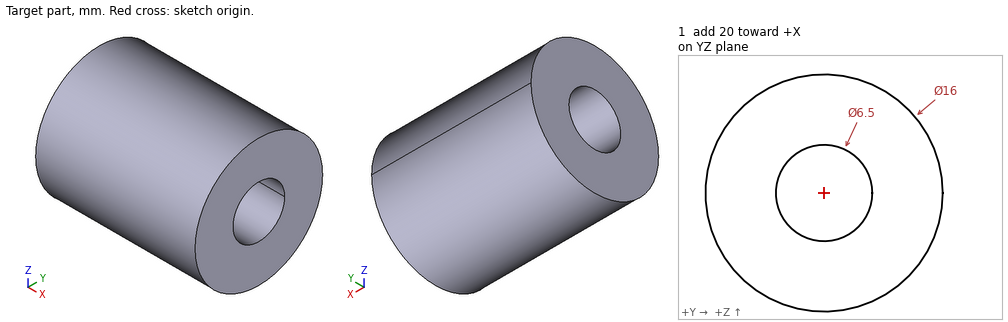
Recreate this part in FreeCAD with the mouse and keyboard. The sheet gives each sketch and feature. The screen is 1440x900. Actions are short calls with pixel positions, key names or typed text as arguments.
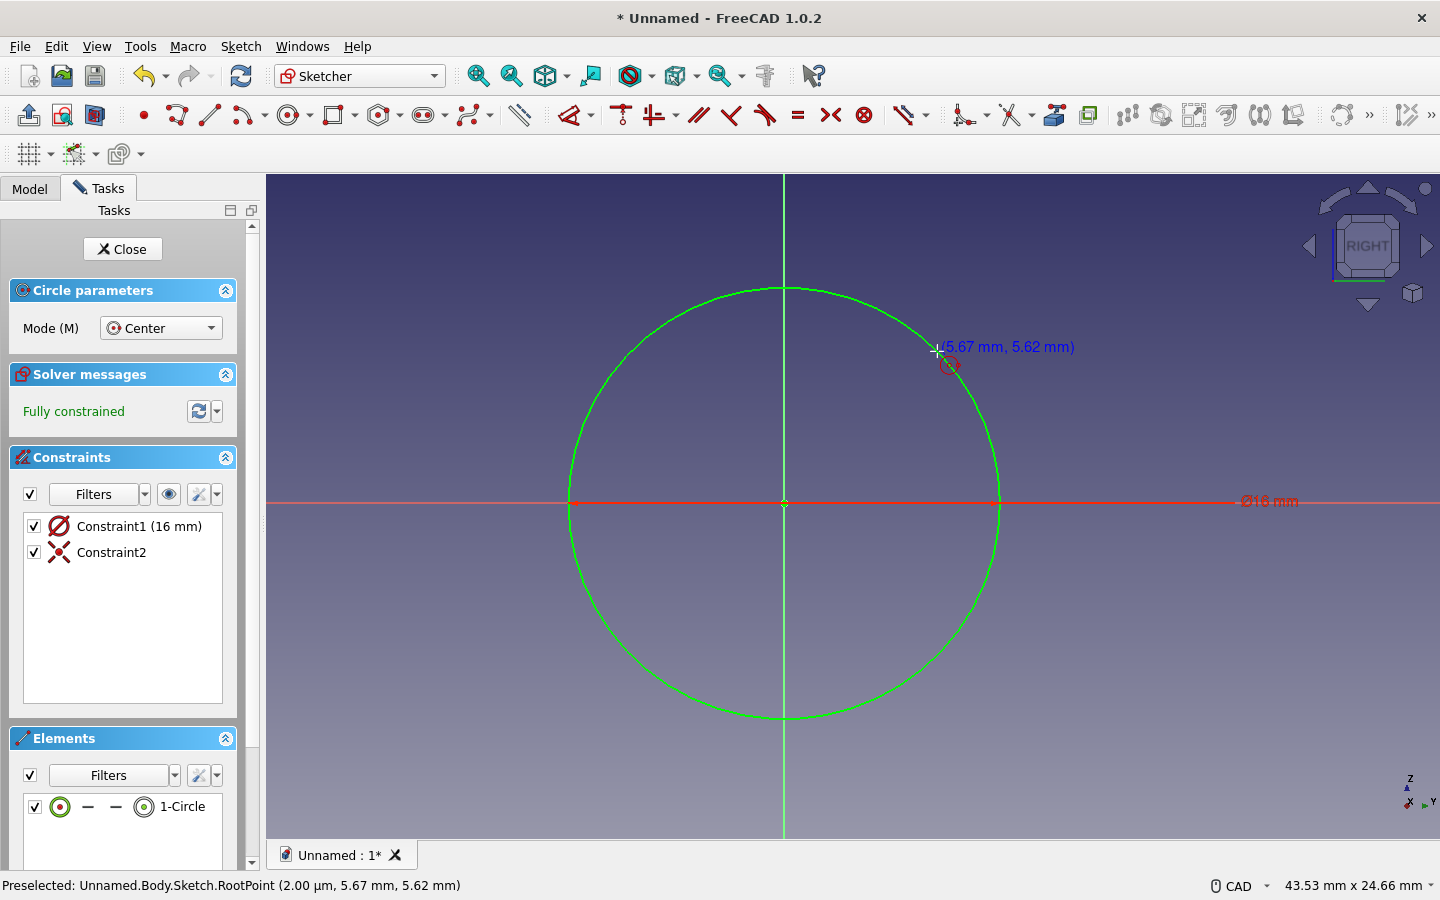
click(784, 503)
move(846, 441)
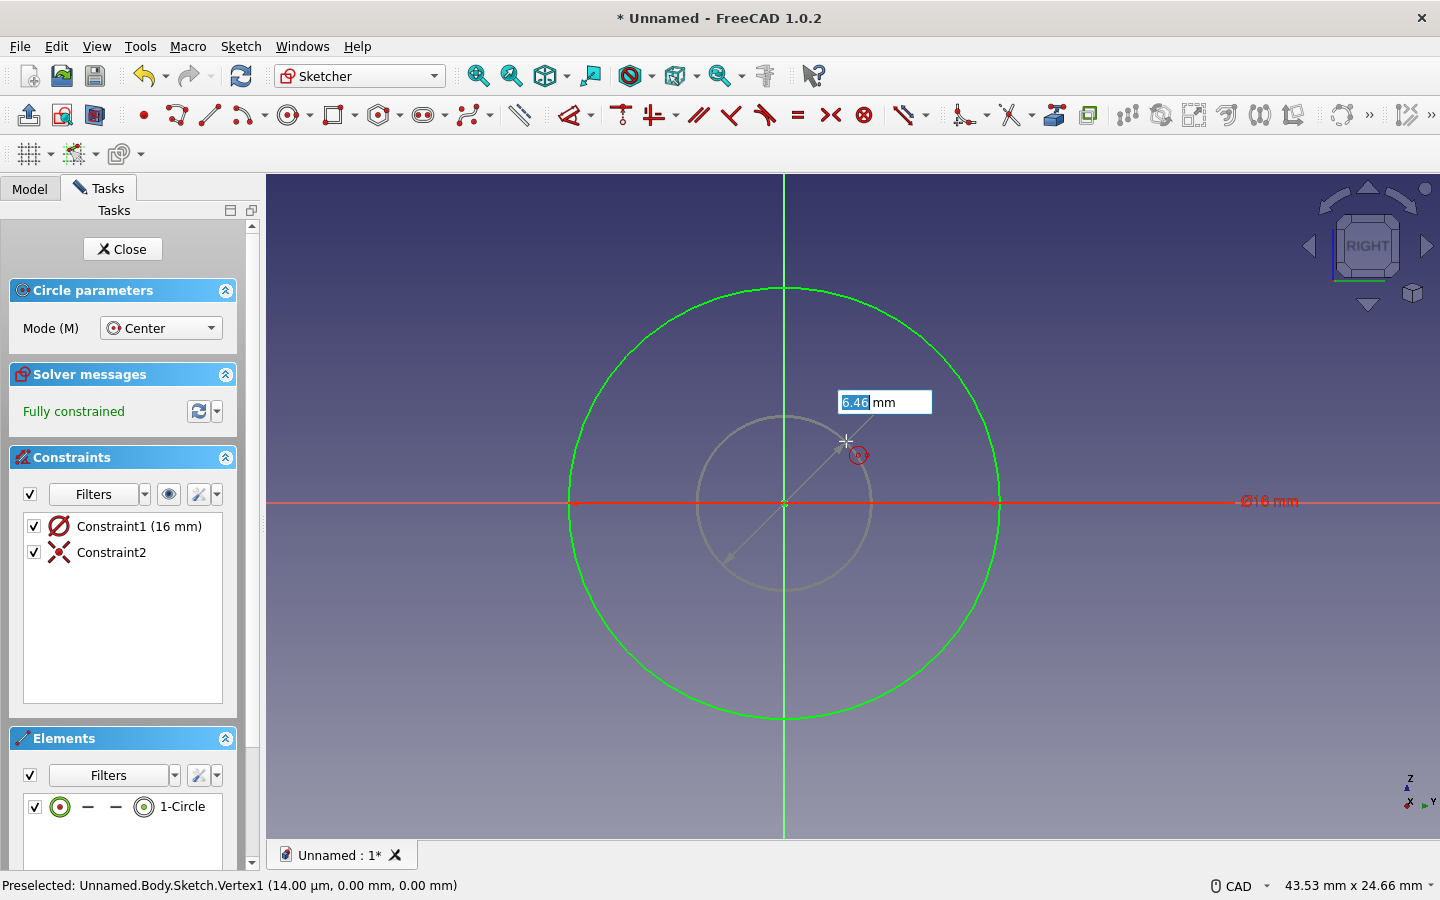
text(6.5)
key(Return)
key(Escape)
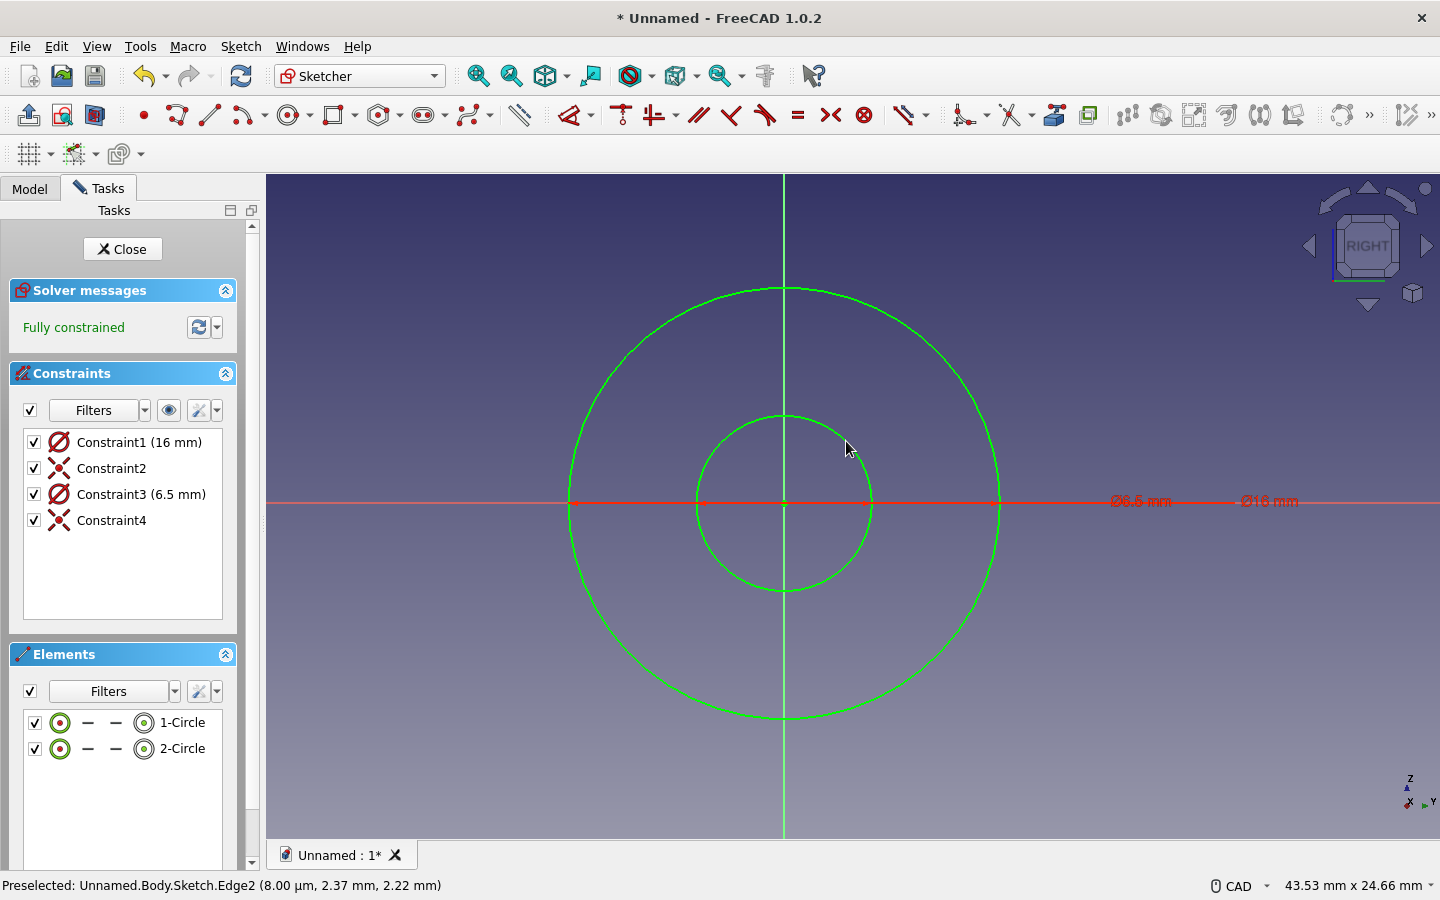
click(123, 249)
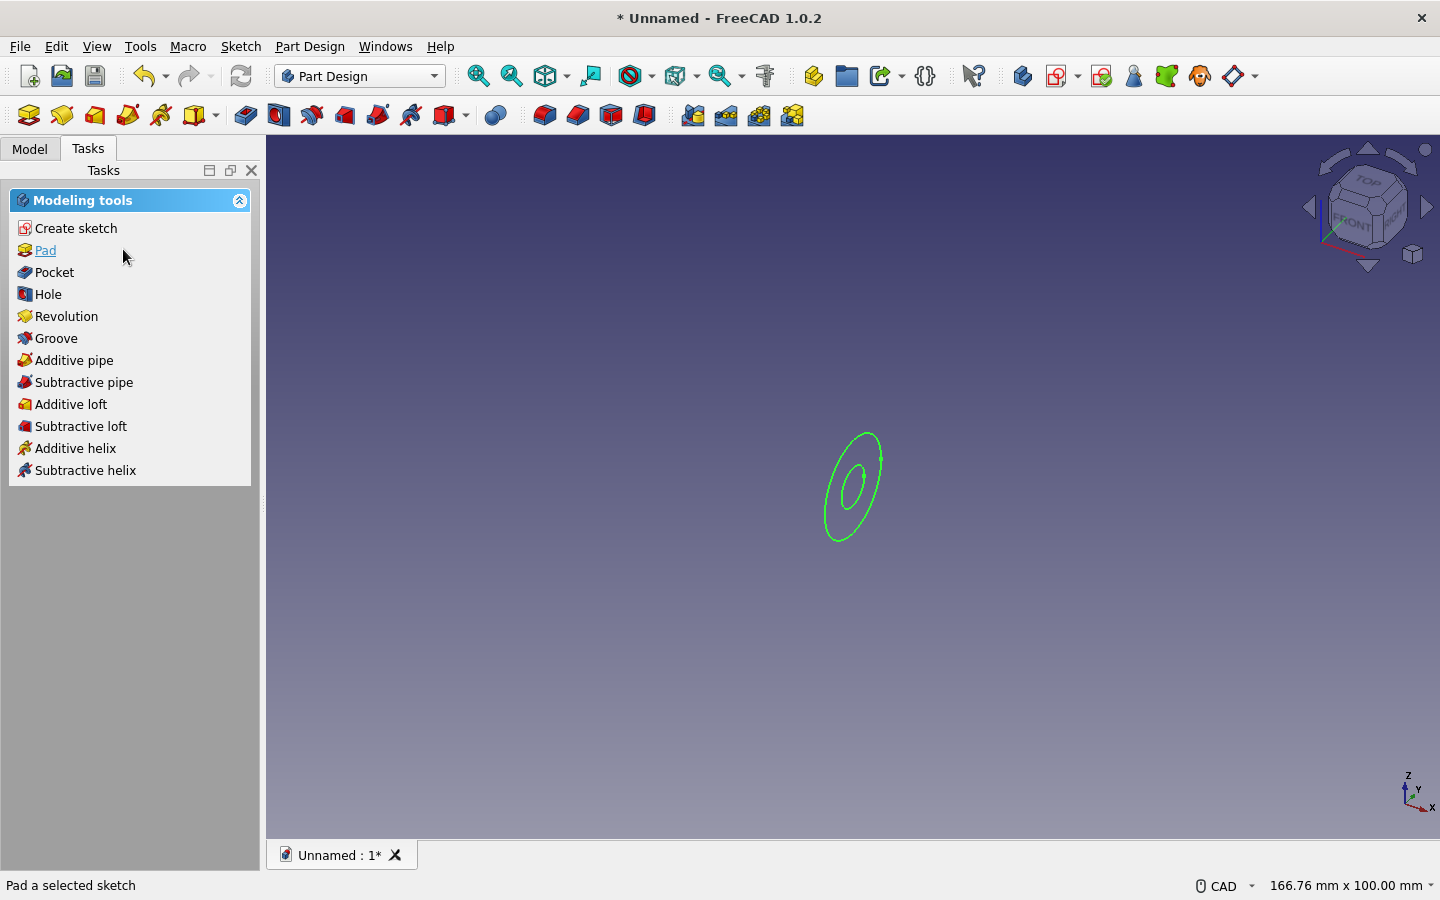
click(29, 116)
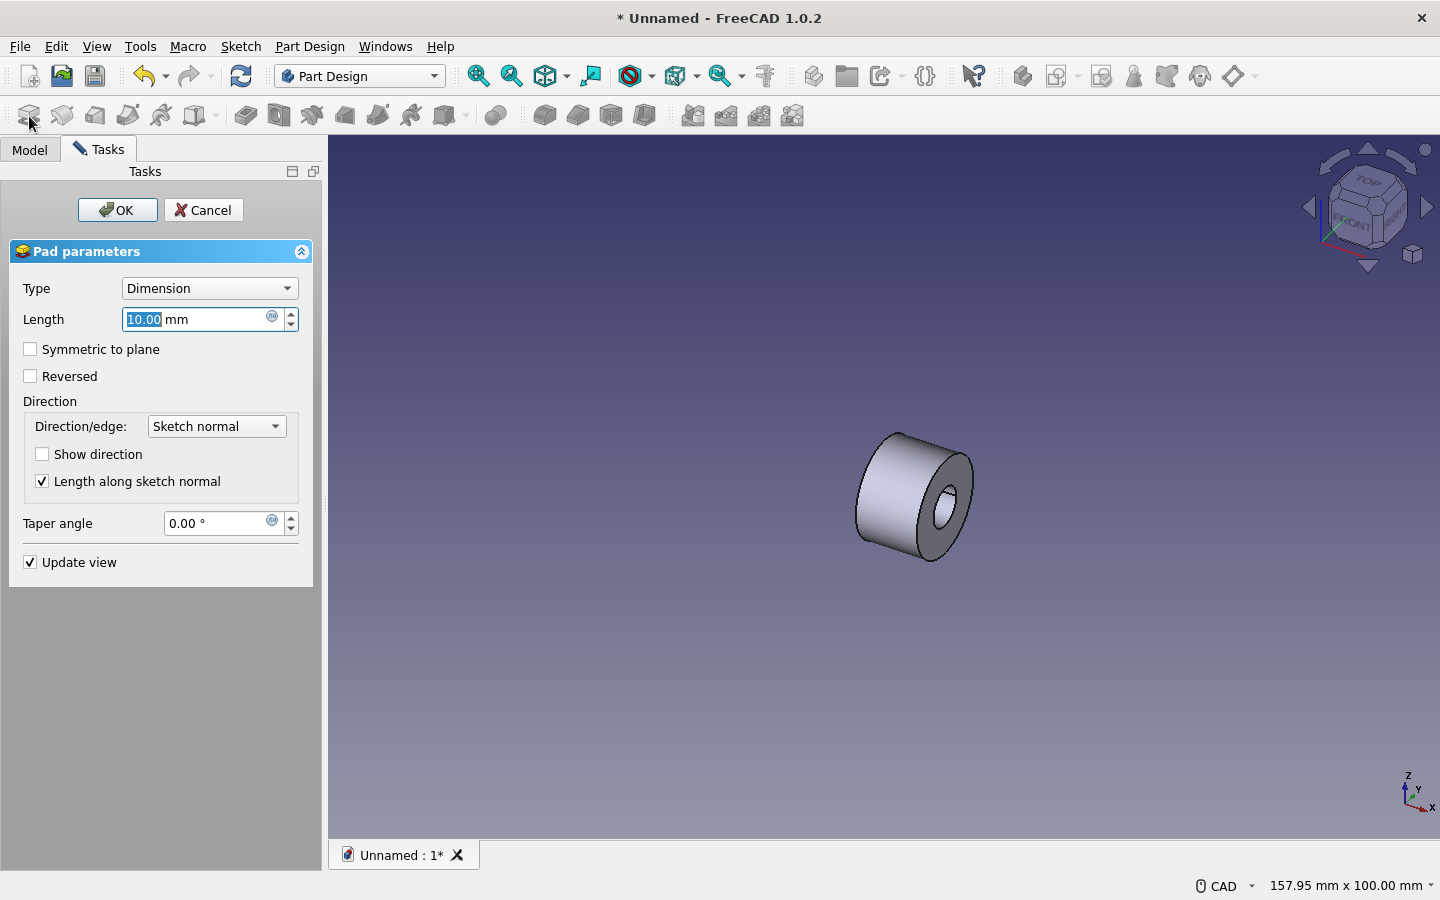
text(20)
key(Tab)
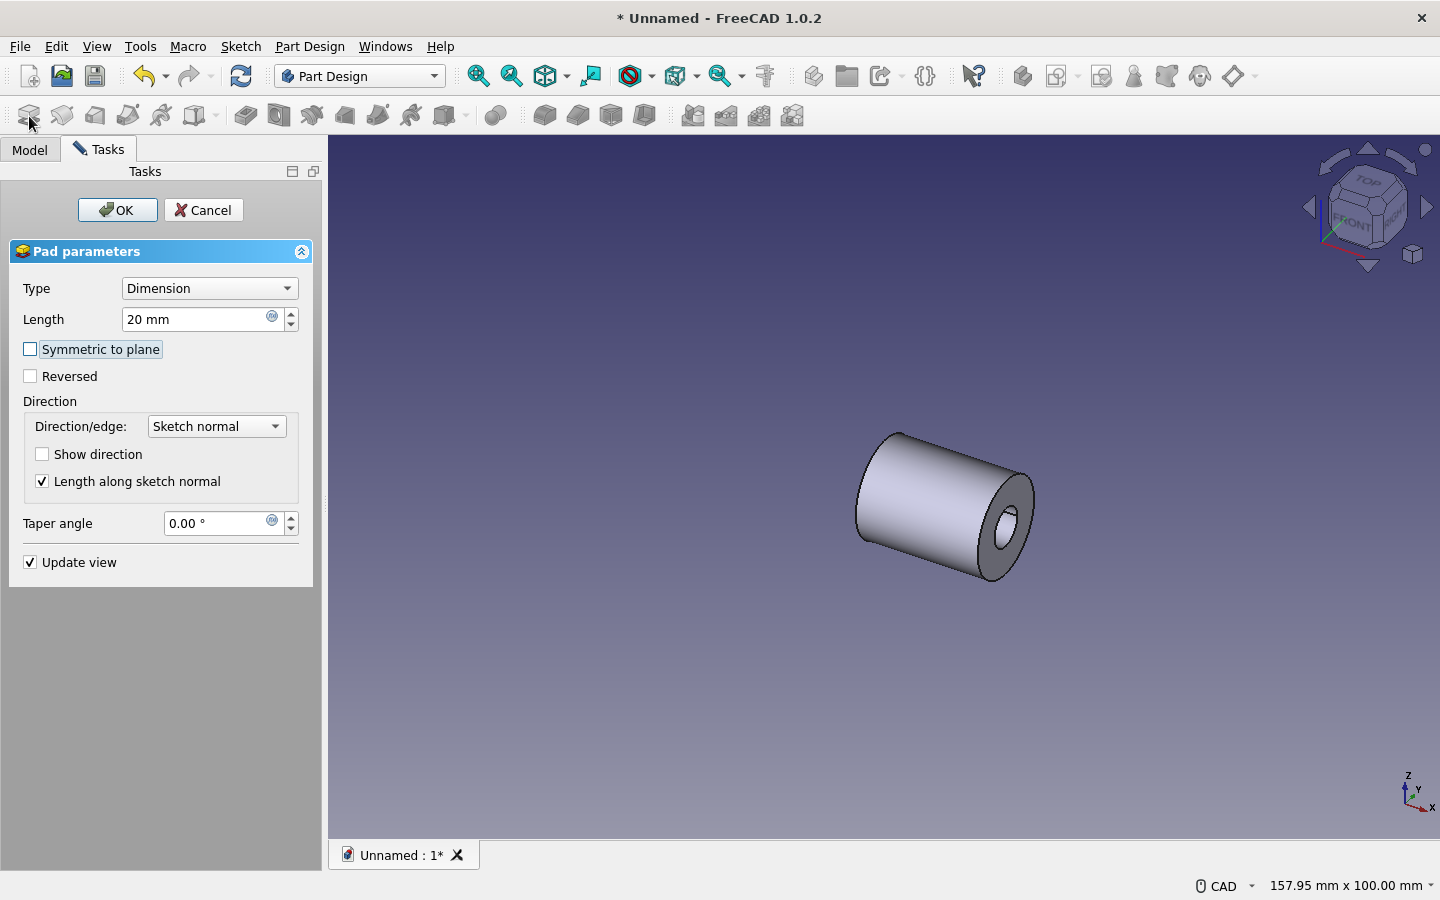
click(118, 210)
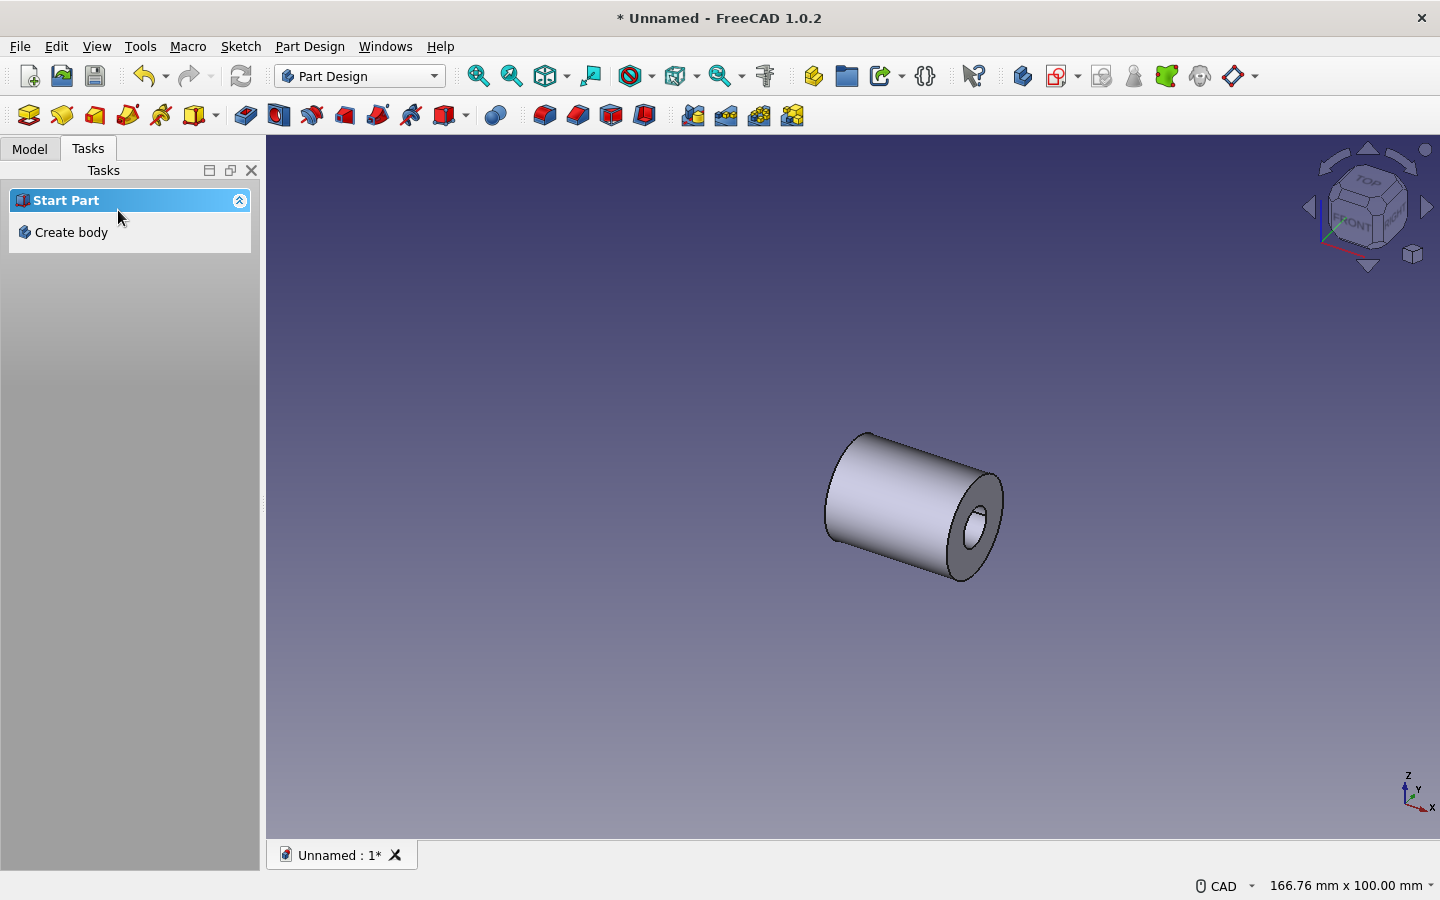
key(0)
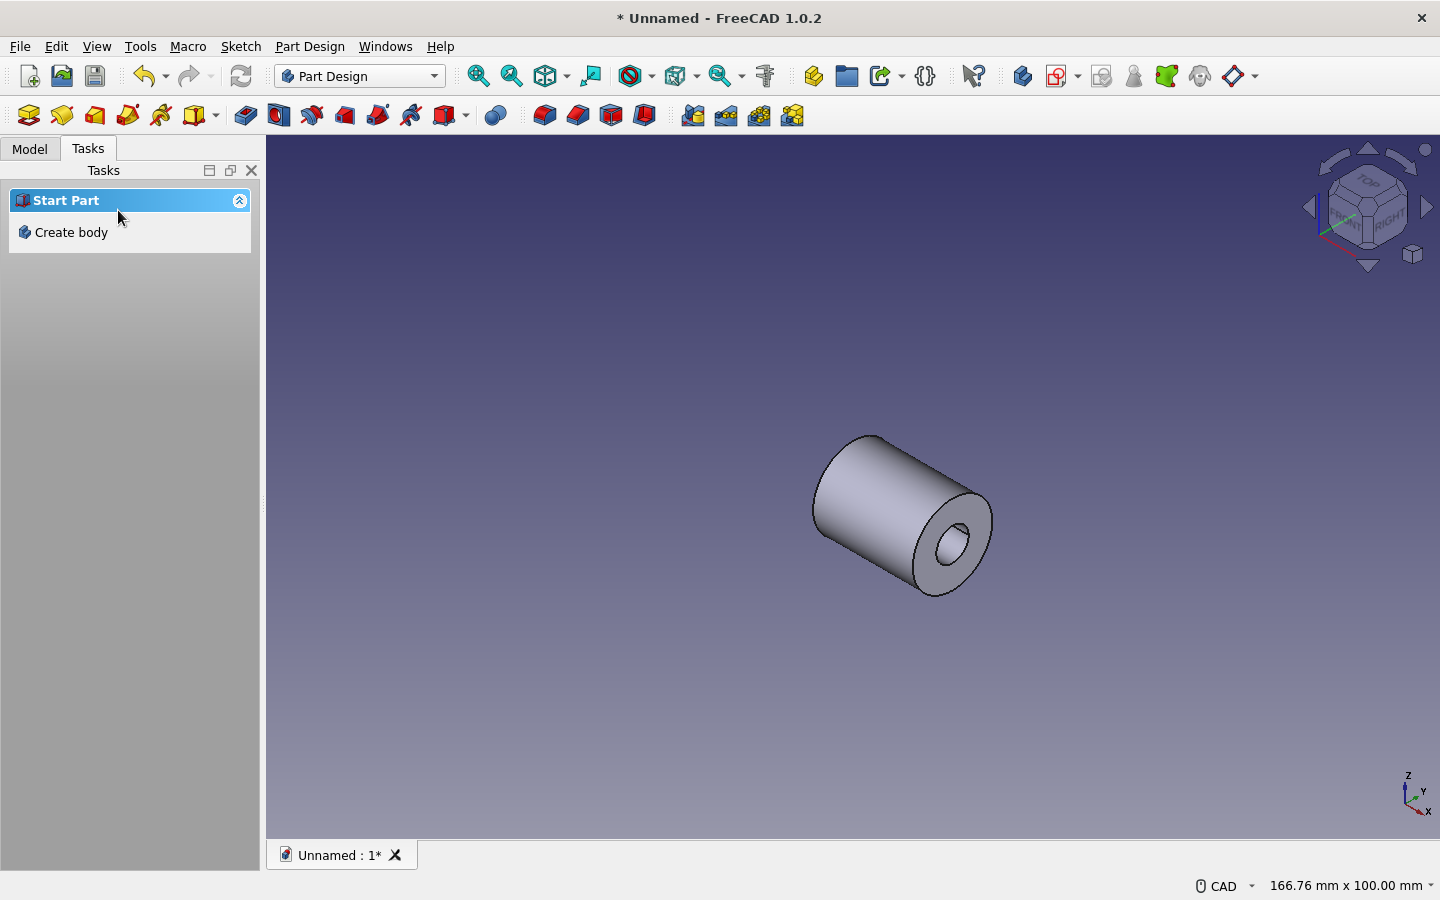
click(479, 76)